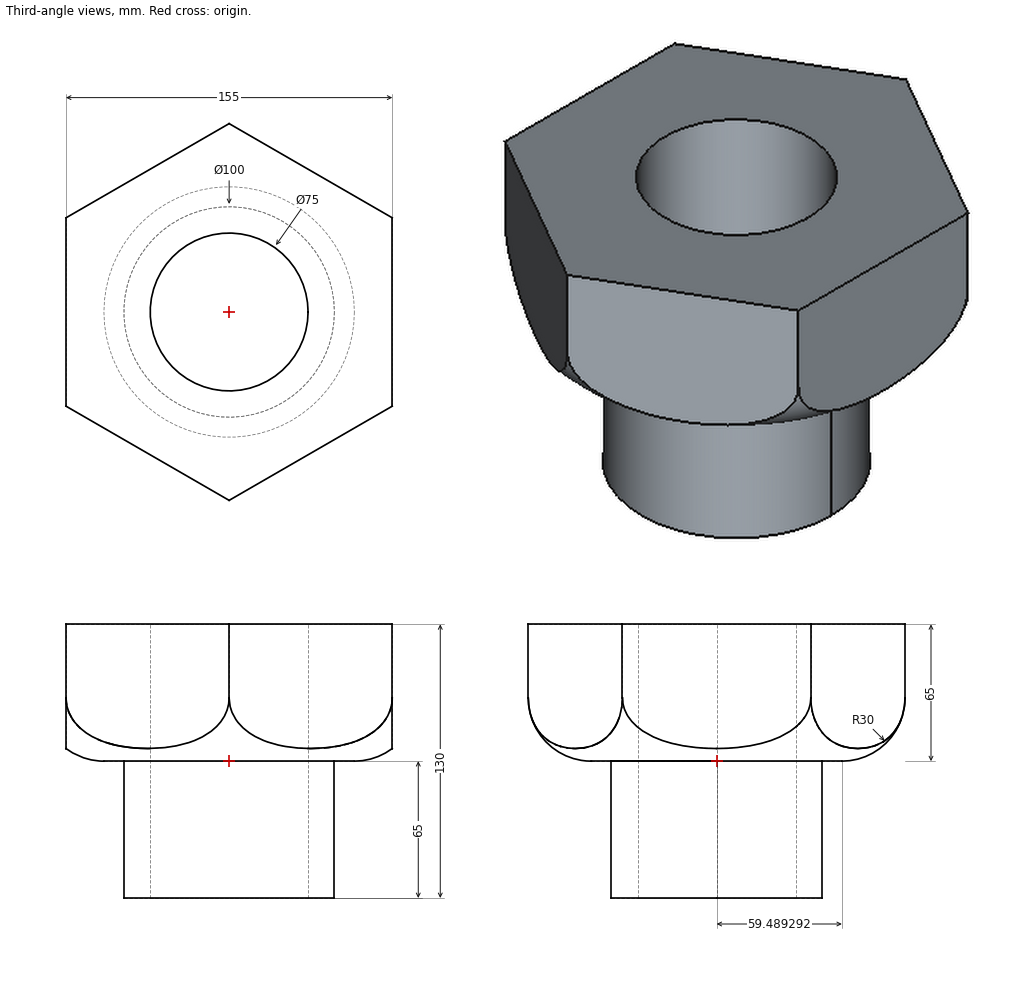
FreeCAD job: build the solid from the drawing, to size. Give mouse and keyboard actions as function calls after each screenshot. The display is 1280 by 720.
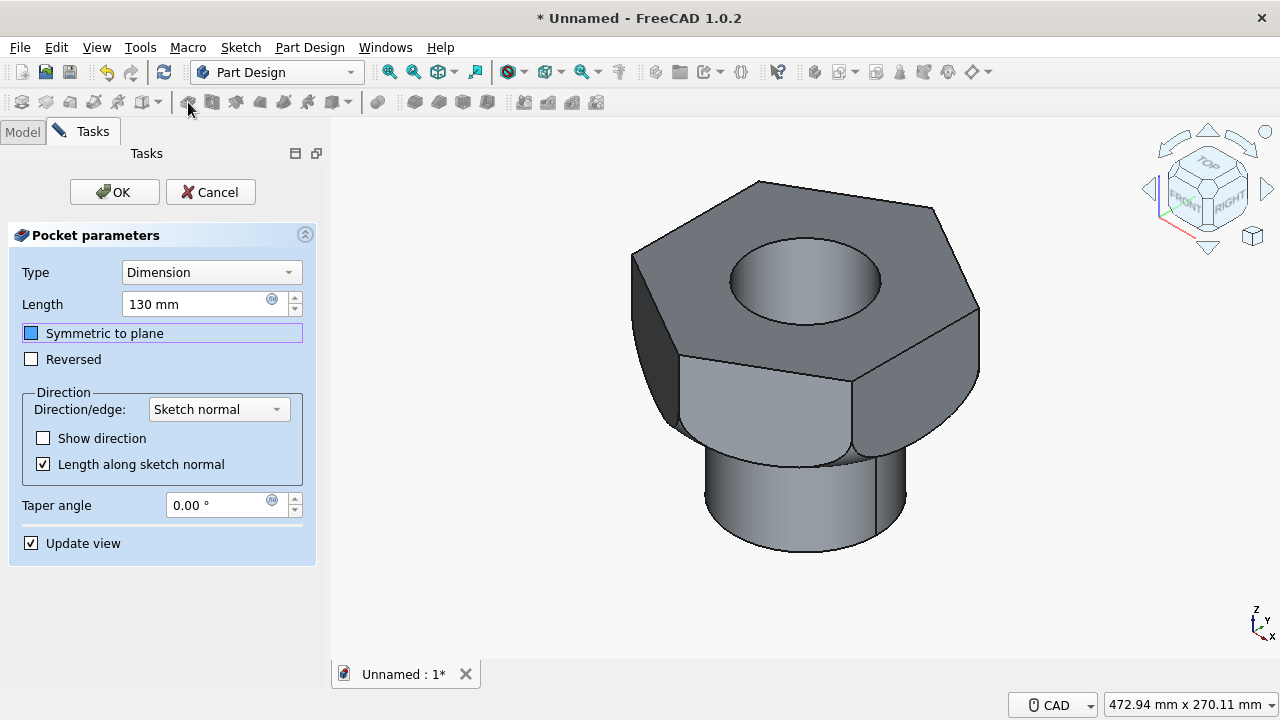
click(115, 192)